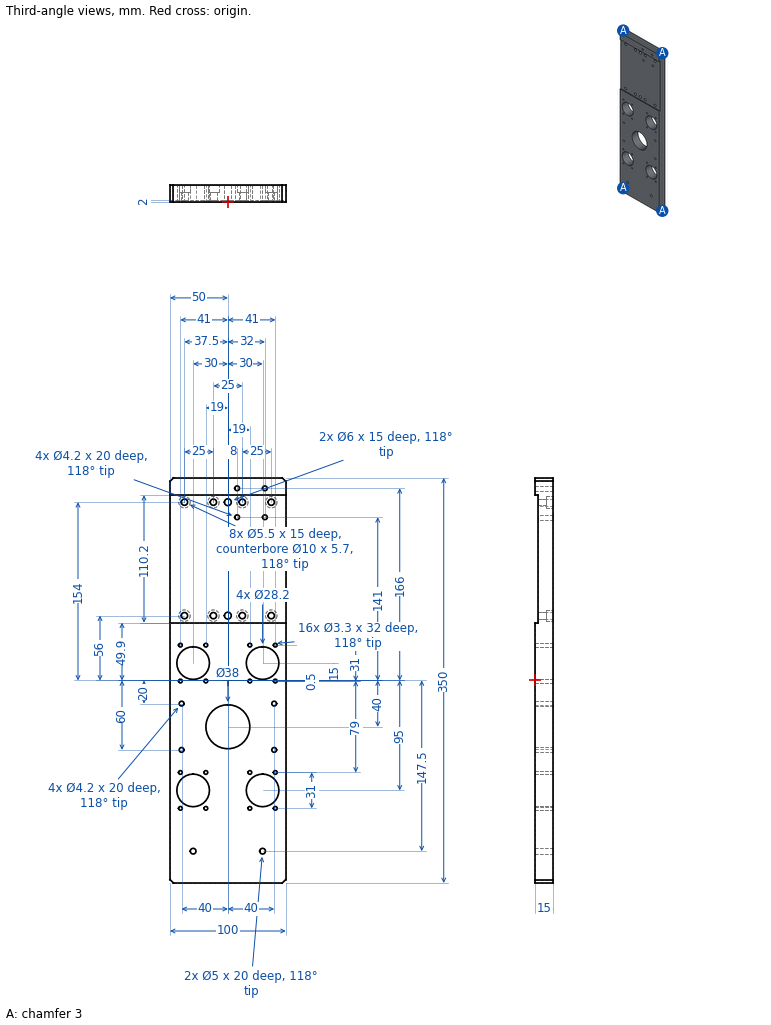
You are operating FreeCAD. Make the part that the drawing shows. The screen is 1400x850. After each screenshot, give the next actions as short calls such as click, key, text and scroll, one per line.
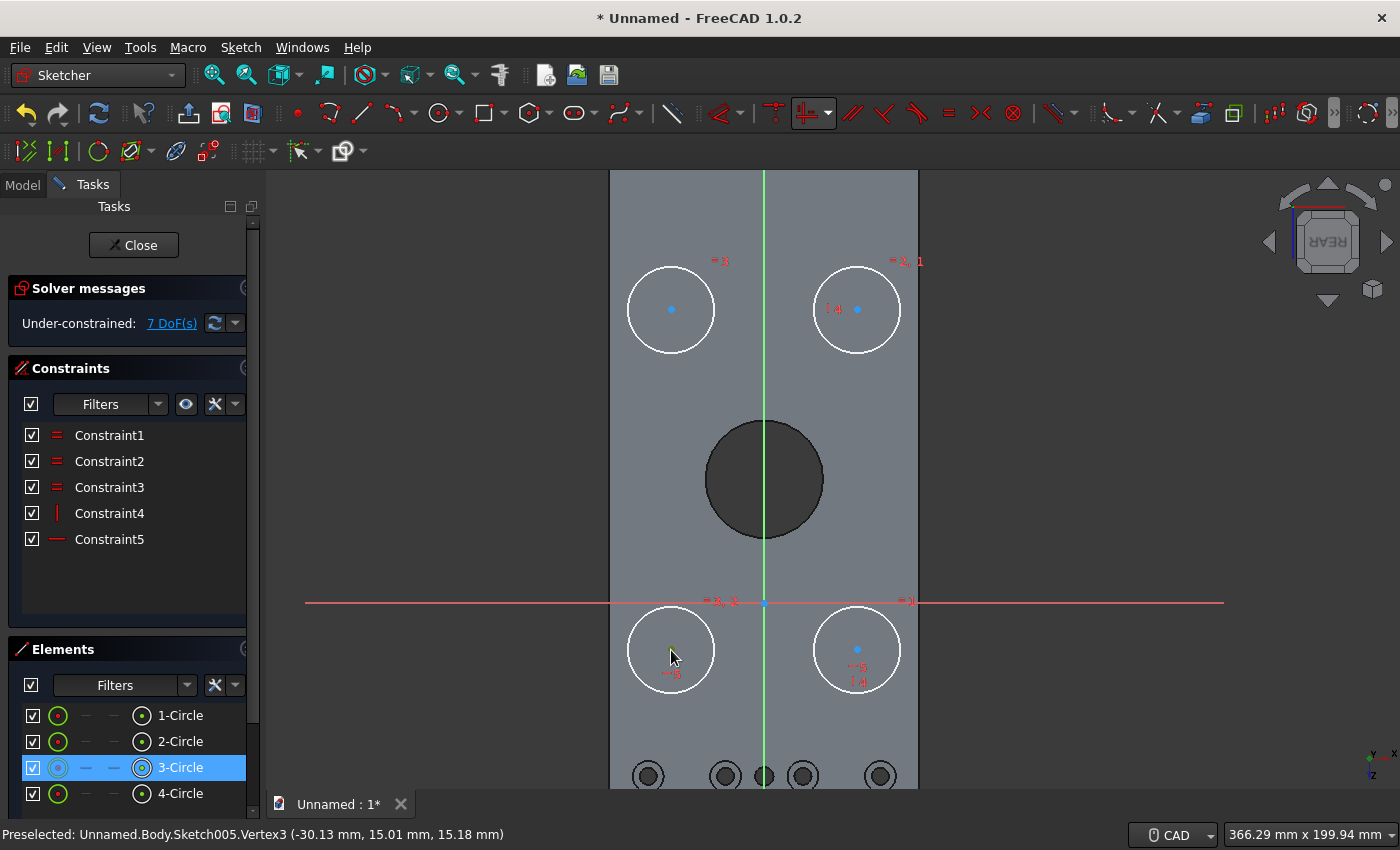
click(671, 310)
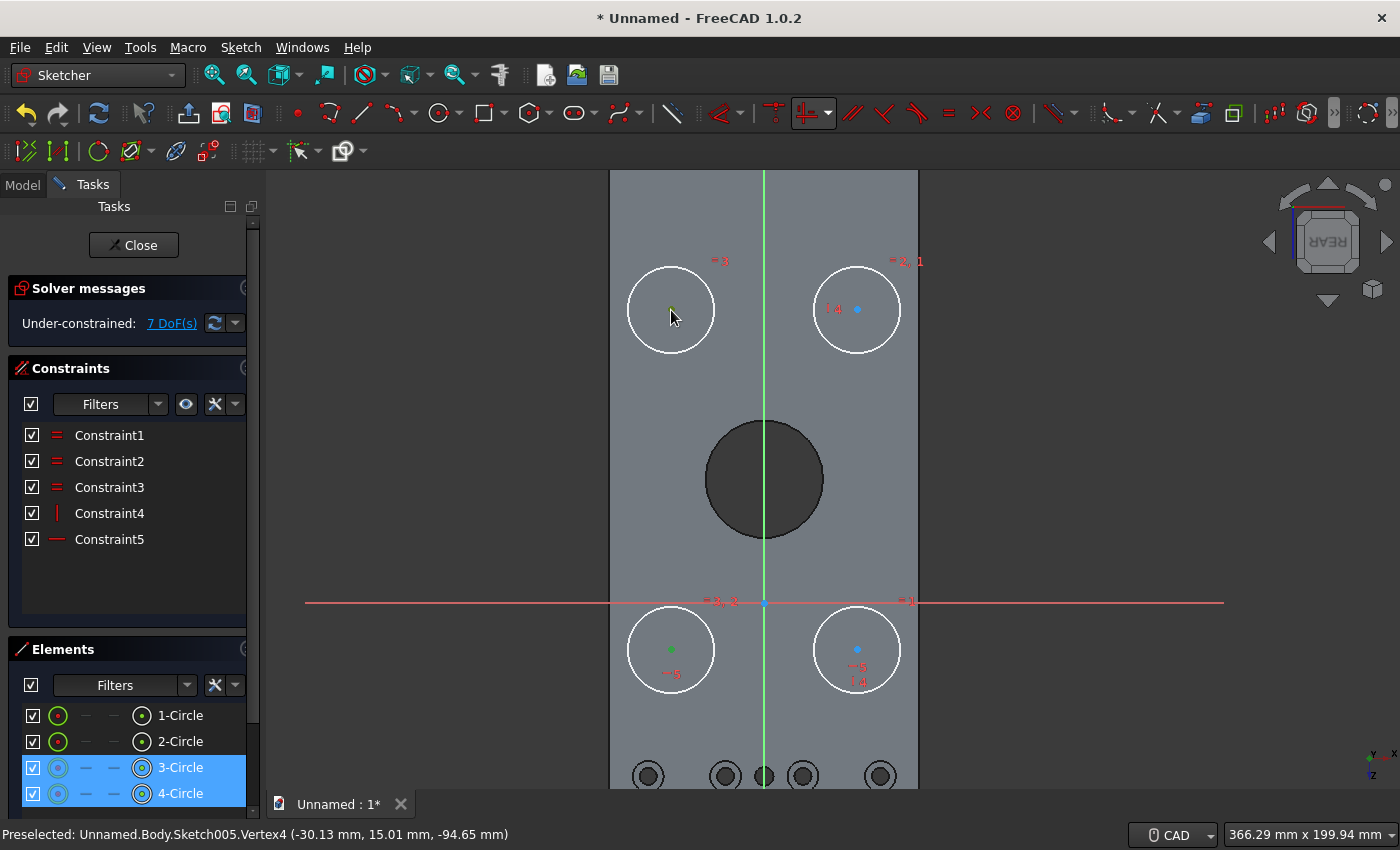
key(v)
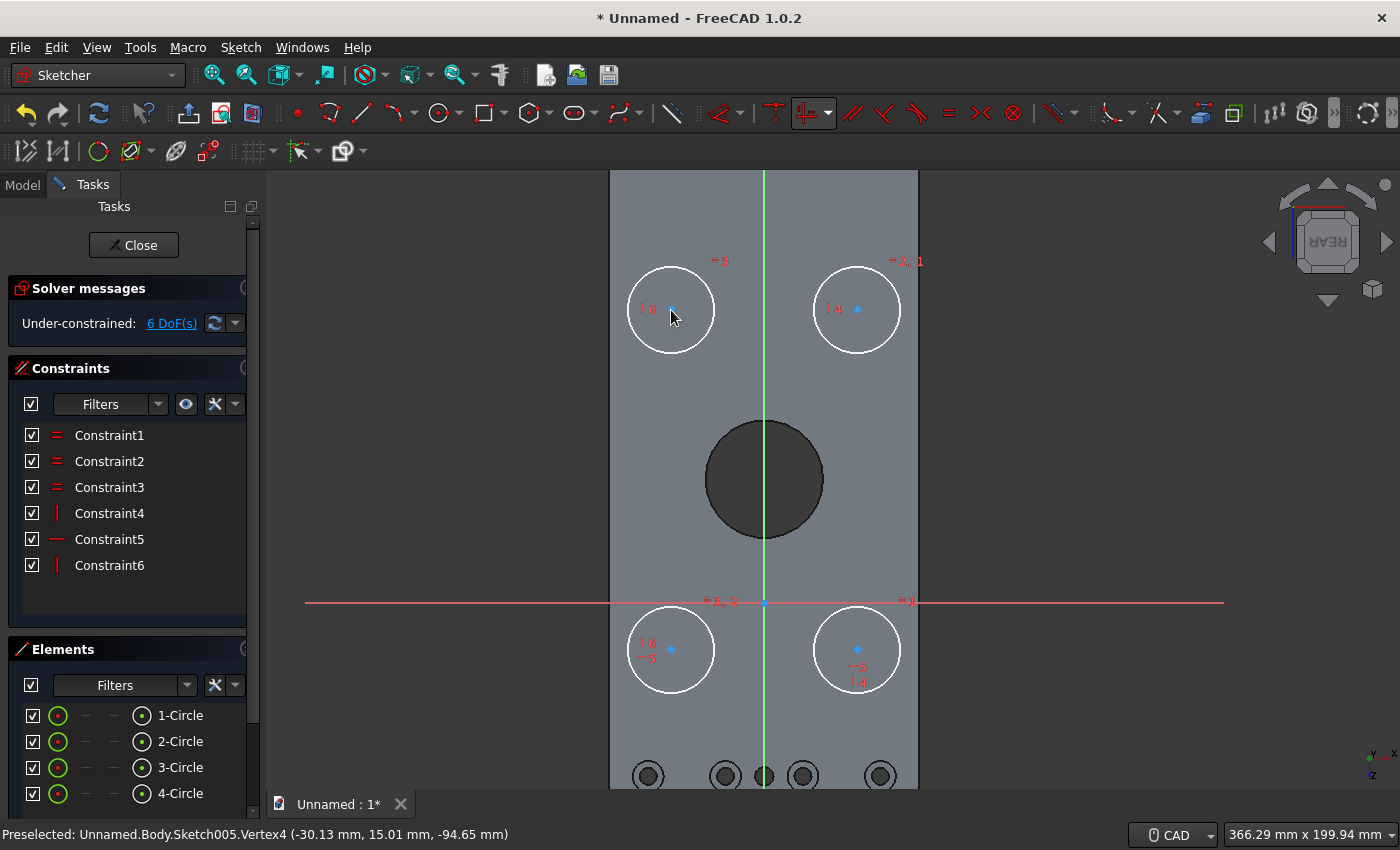
click(857, 310)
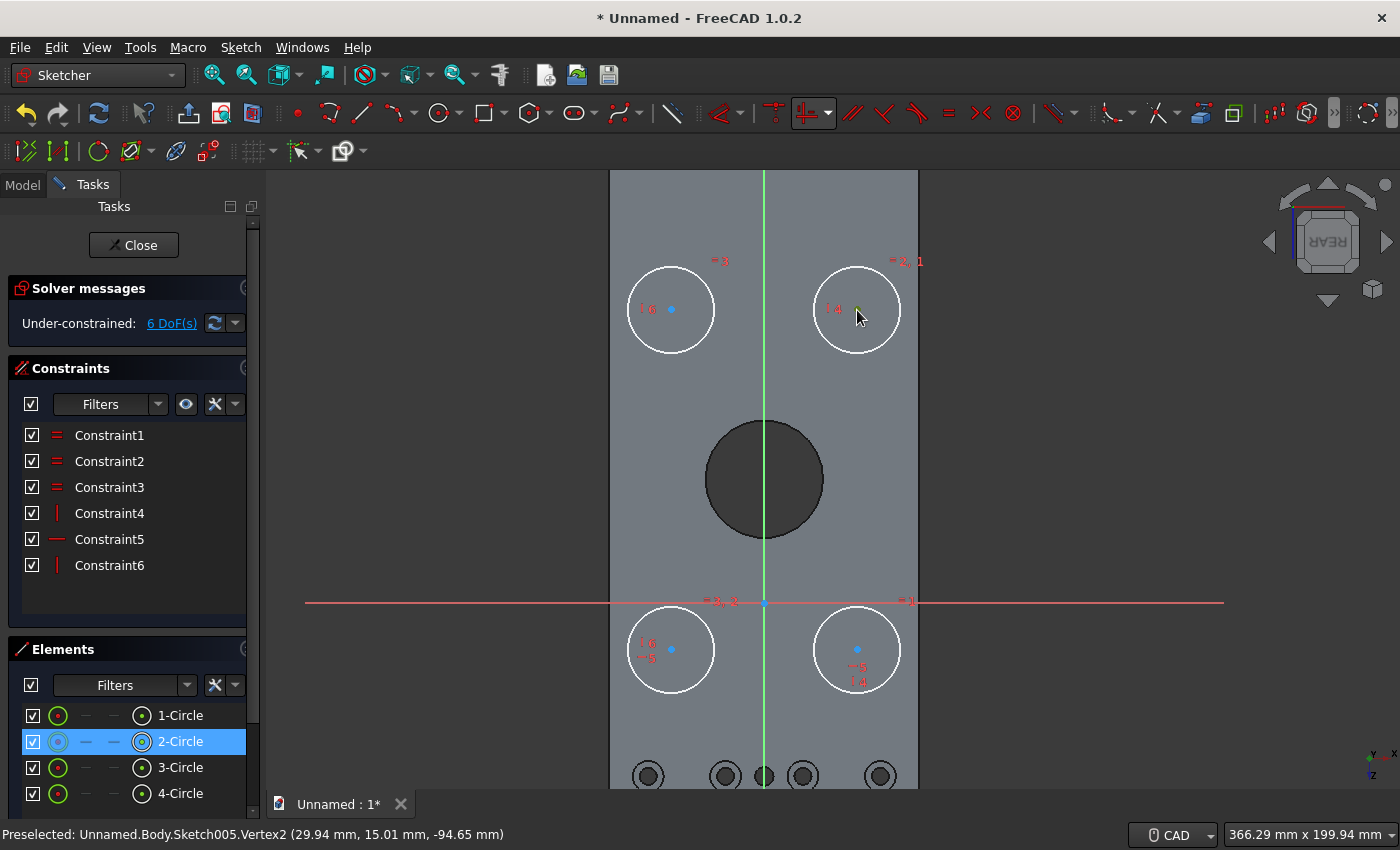
click(671, 310)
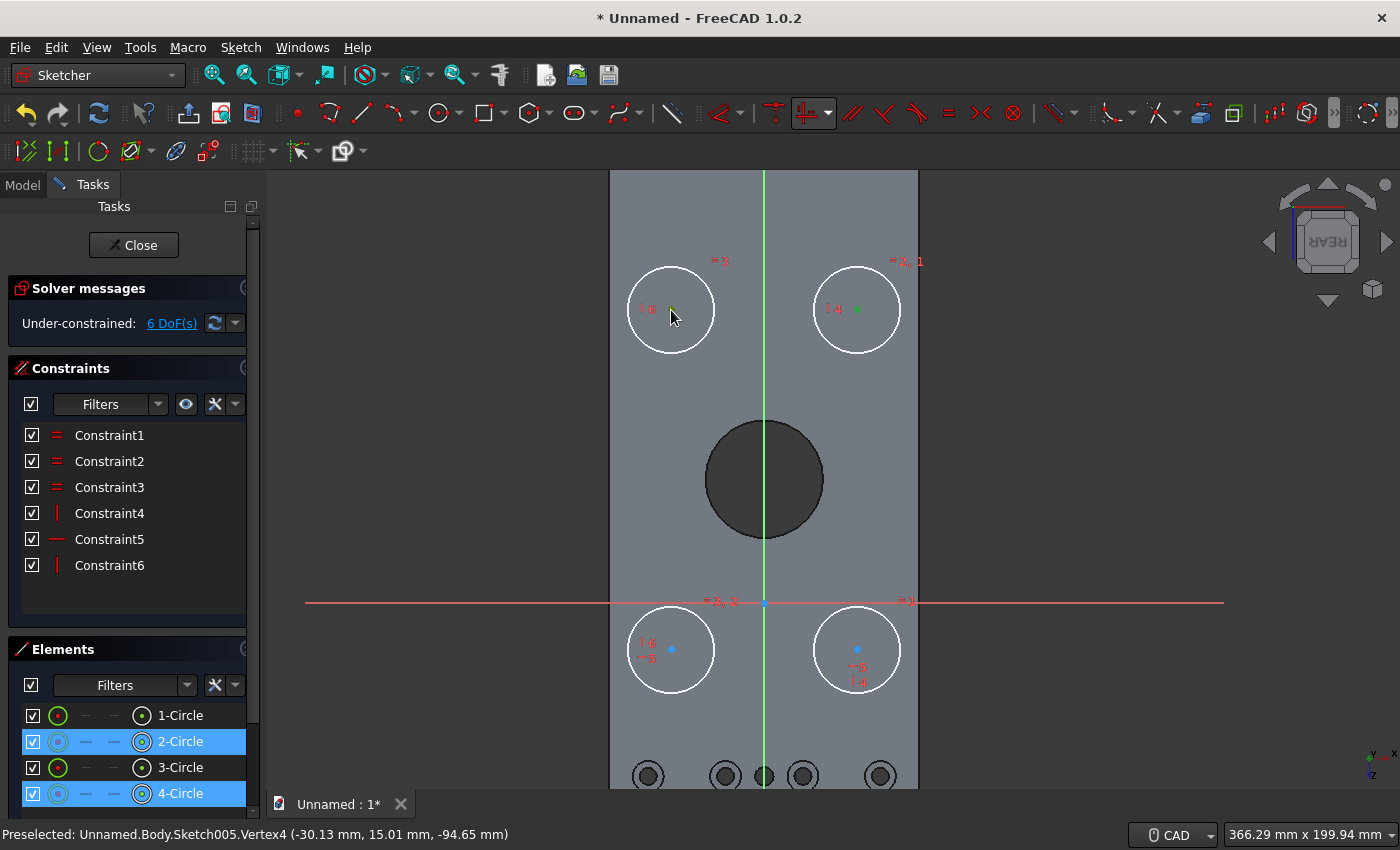
key(h)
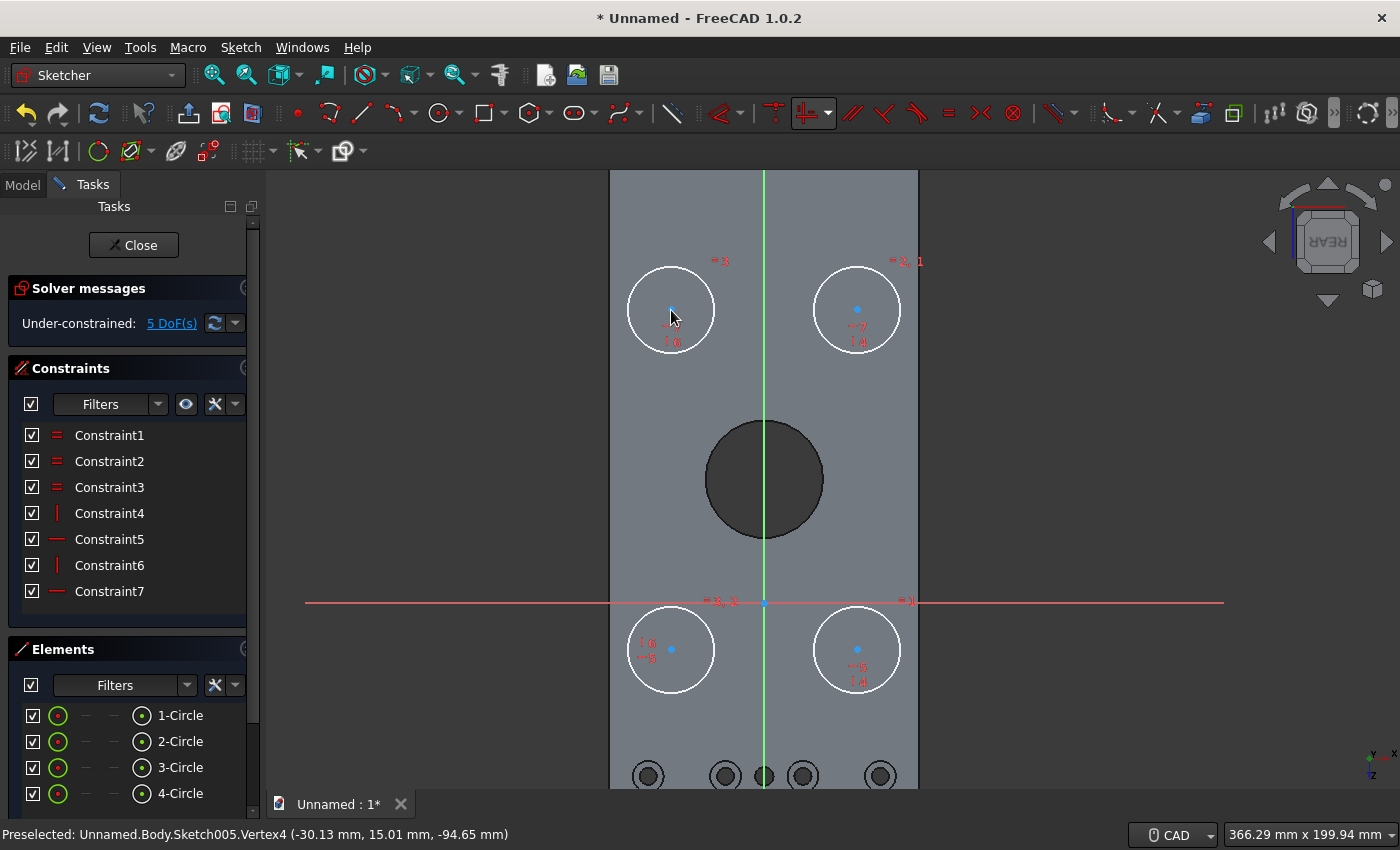
key(d)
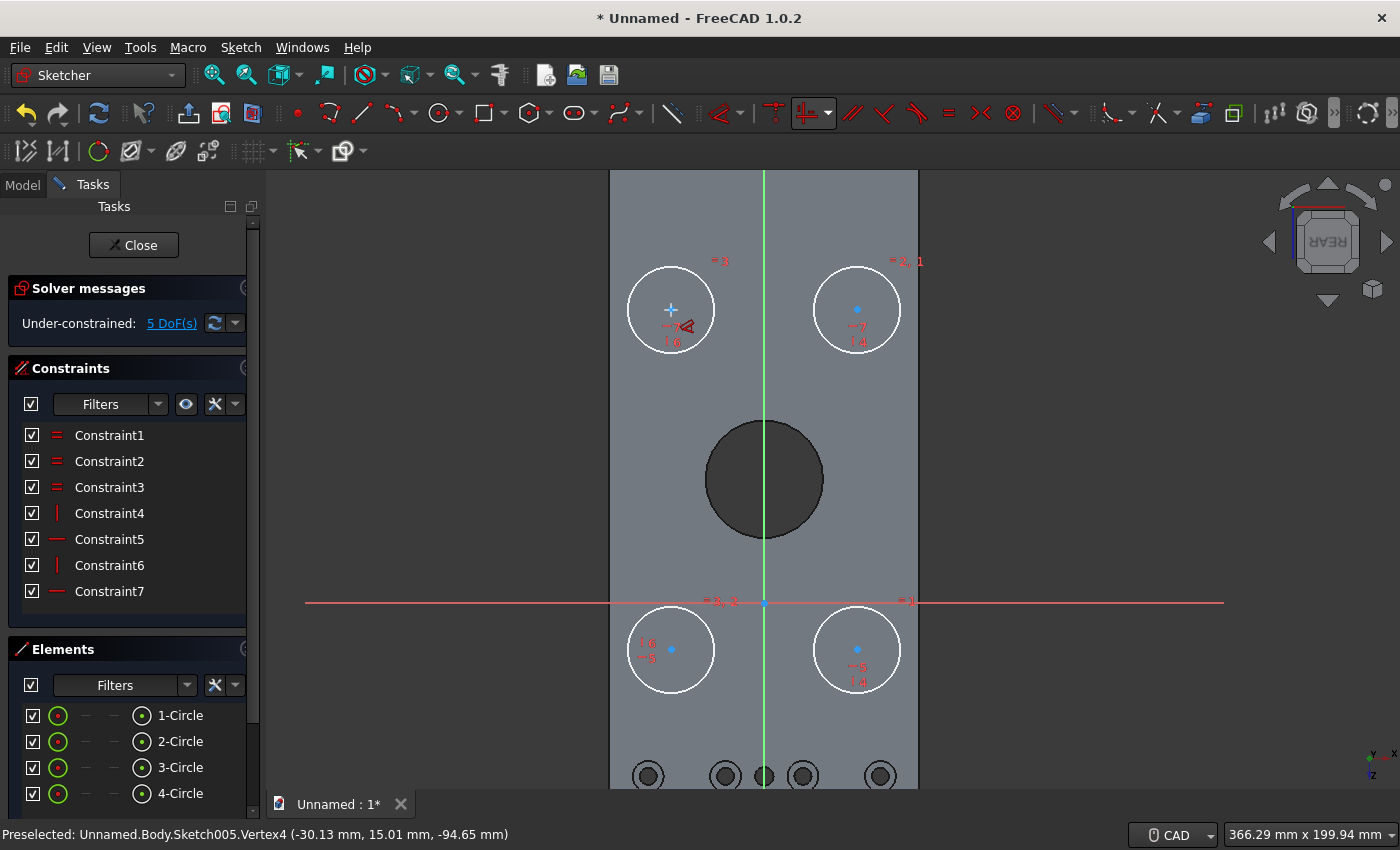
click(887, 619)
click(929, 628)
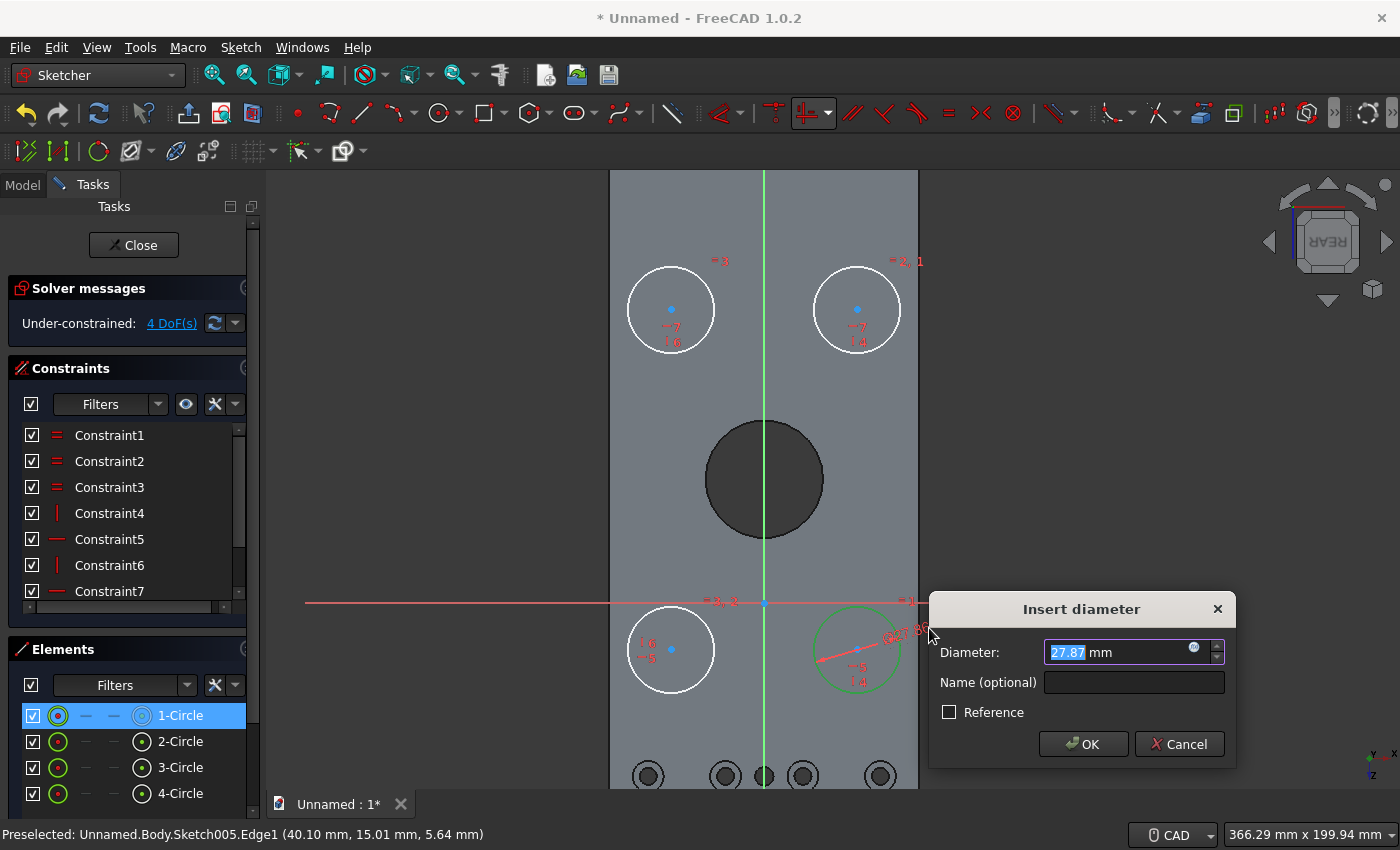
text(28.2)
key(Return)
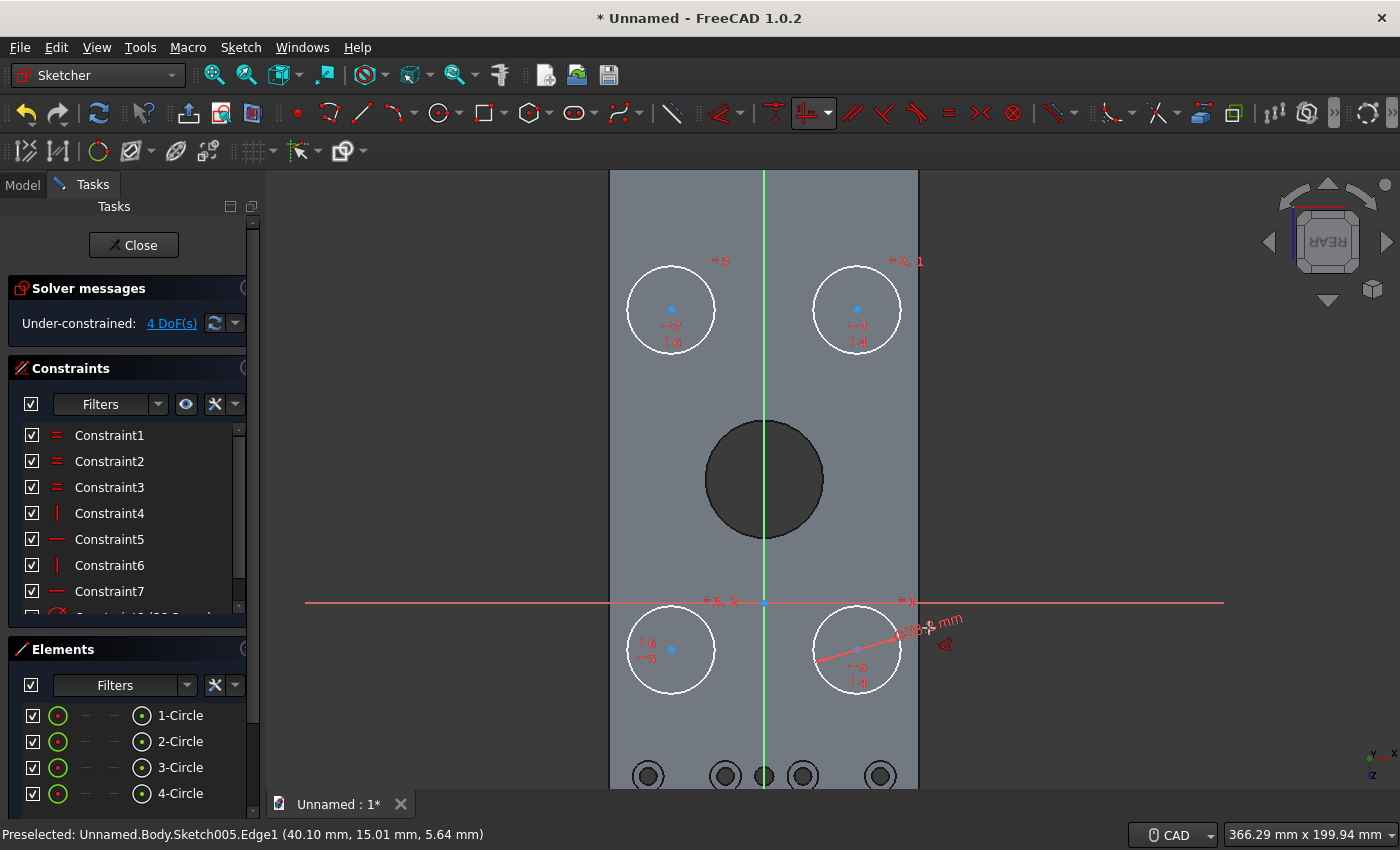
click(857, 650)
click(811, 684)